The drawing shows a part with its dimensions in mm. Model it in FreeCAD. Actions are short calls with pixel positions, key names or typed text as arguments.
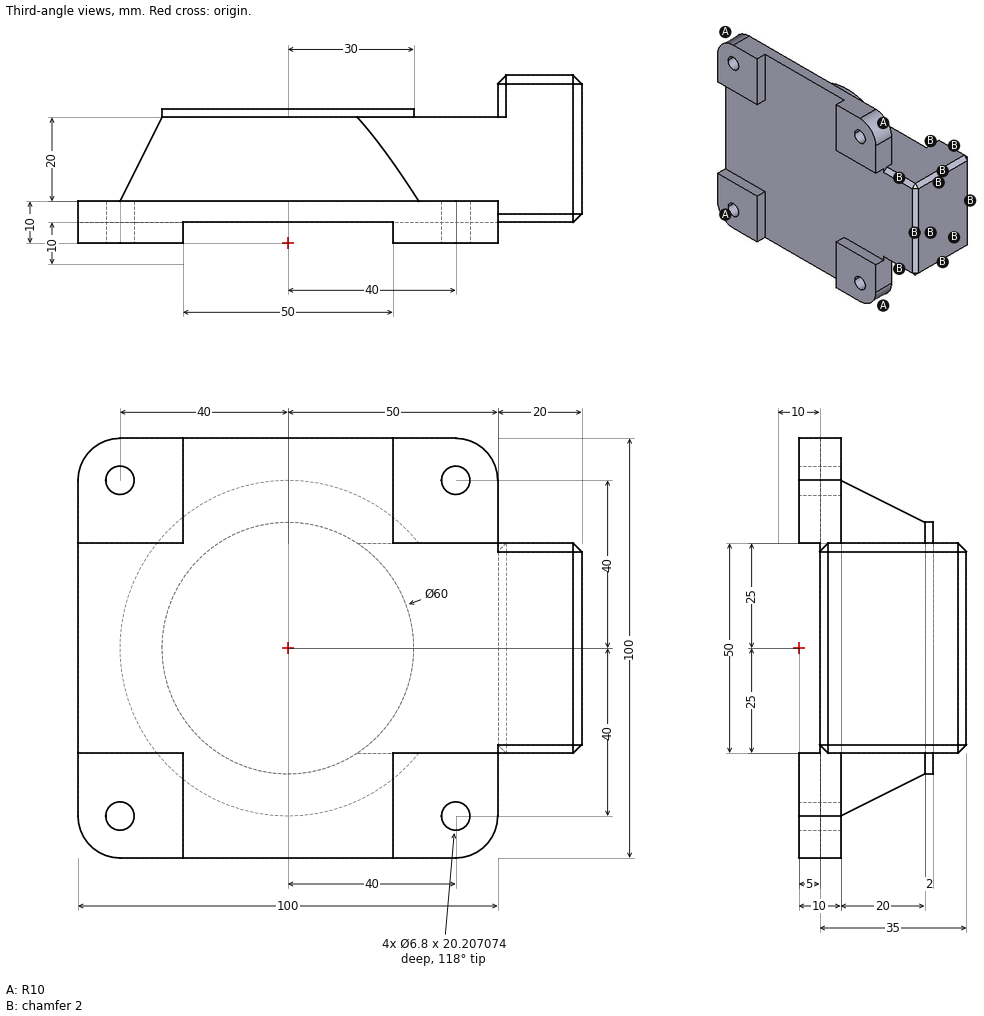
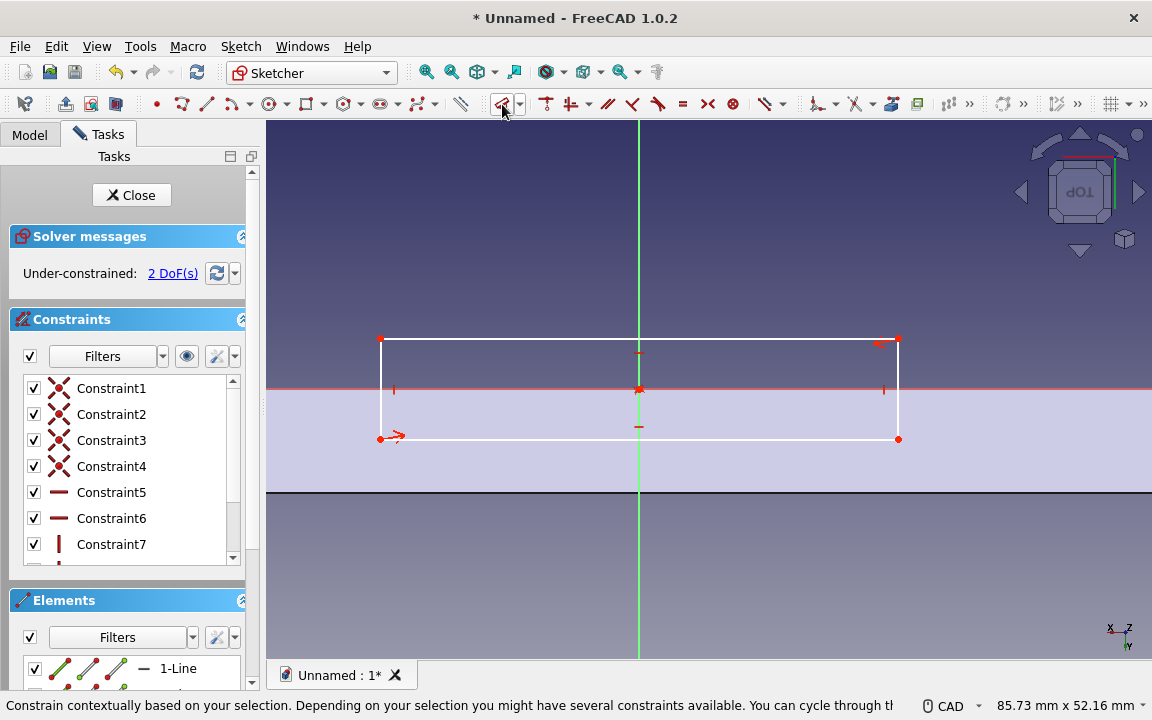
click(536, 440)
click(520, 474)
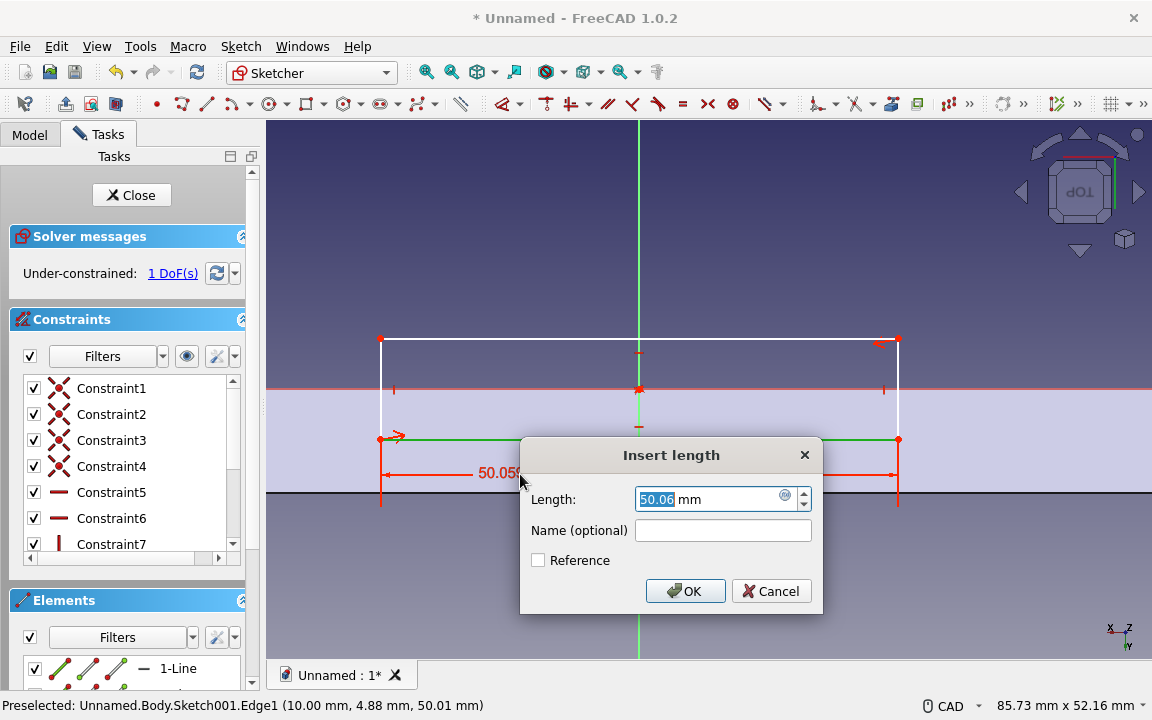
text(50)
key(Return)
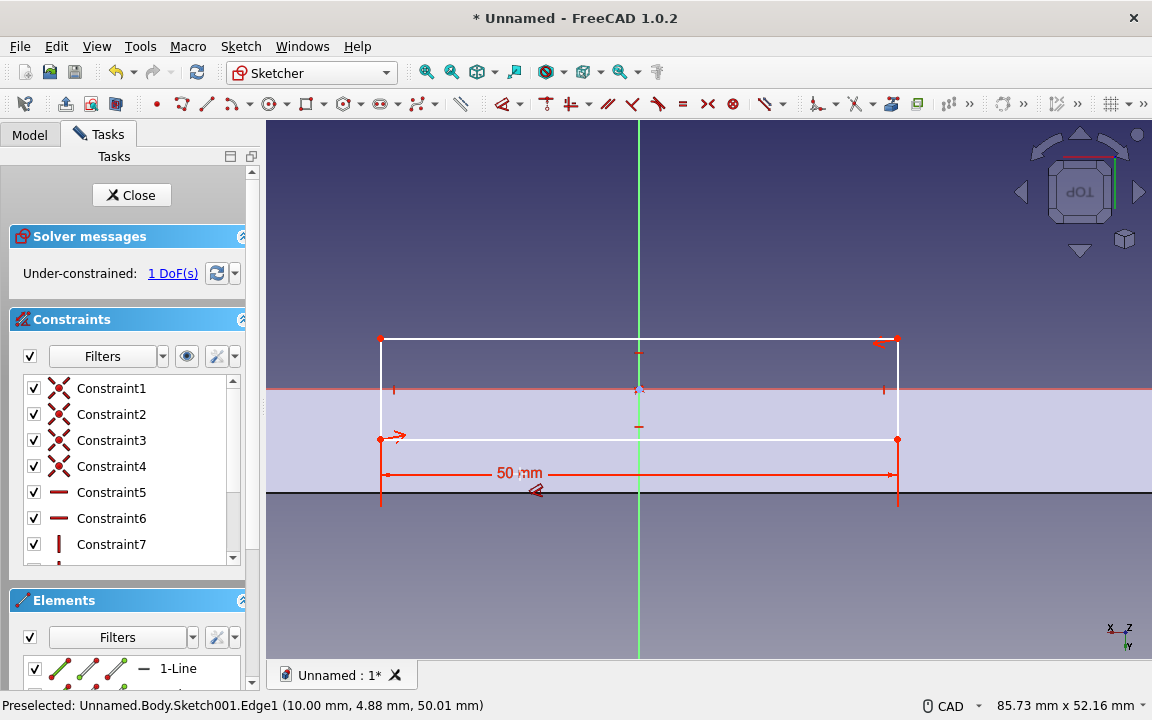
click(898, 410)
click(932, 366)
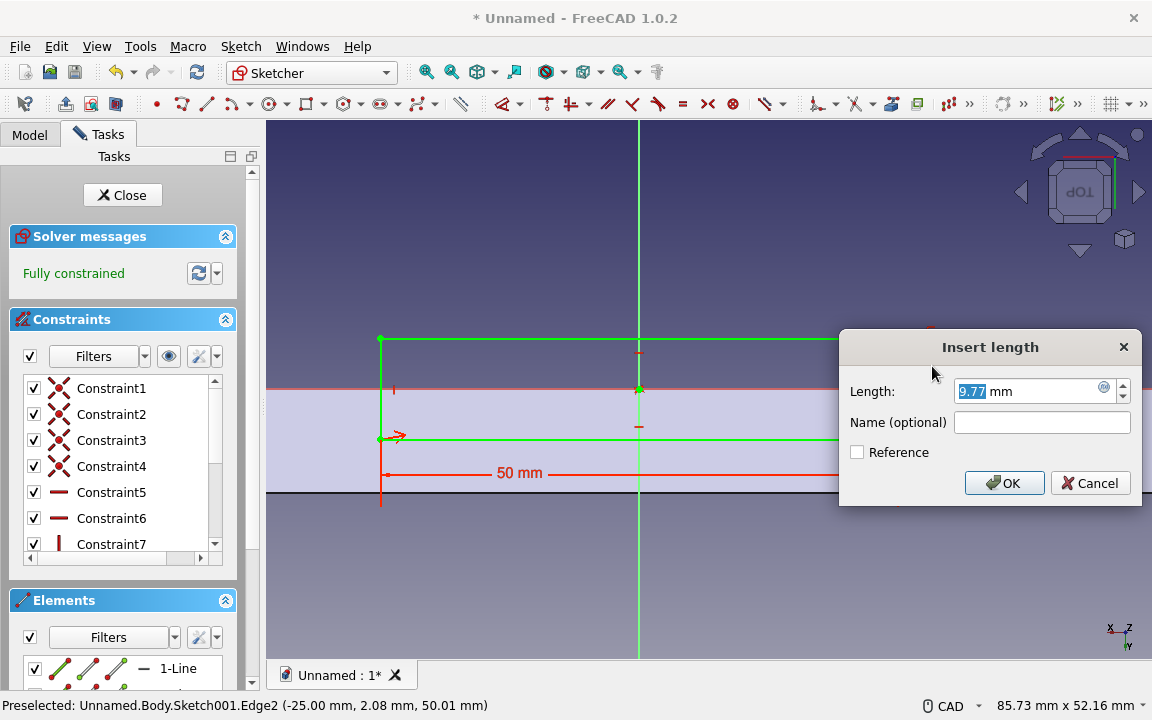
text(10)
key(Return)
key(Escape)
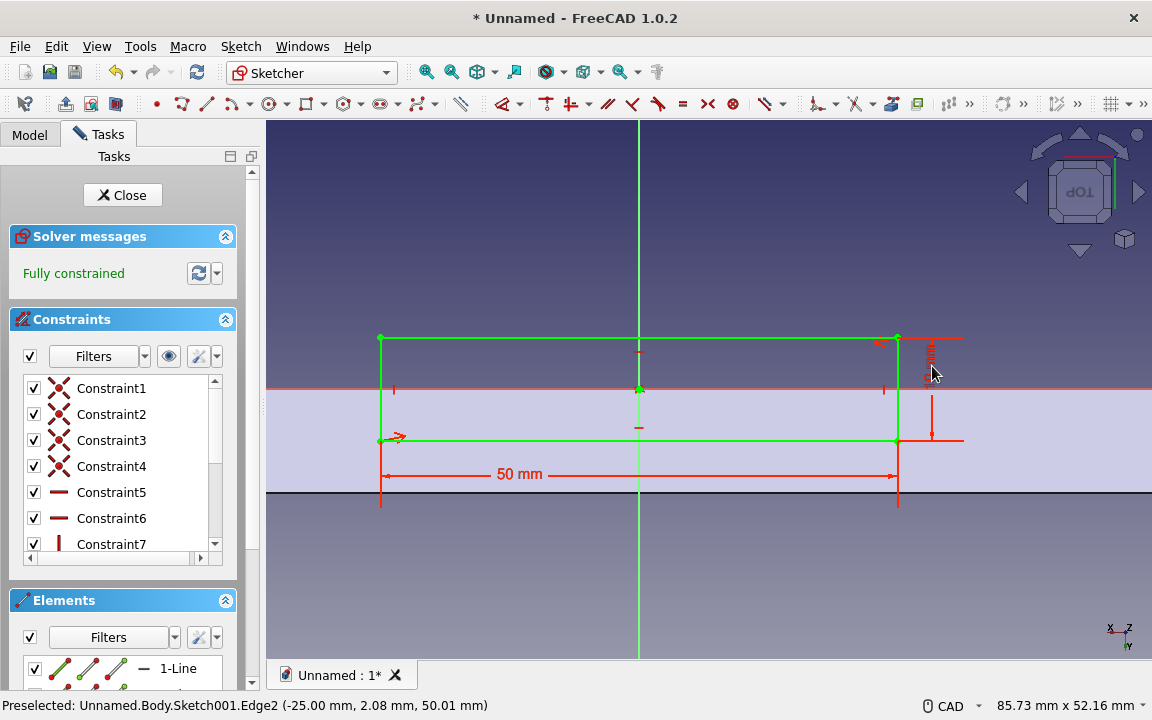
click(123, 195)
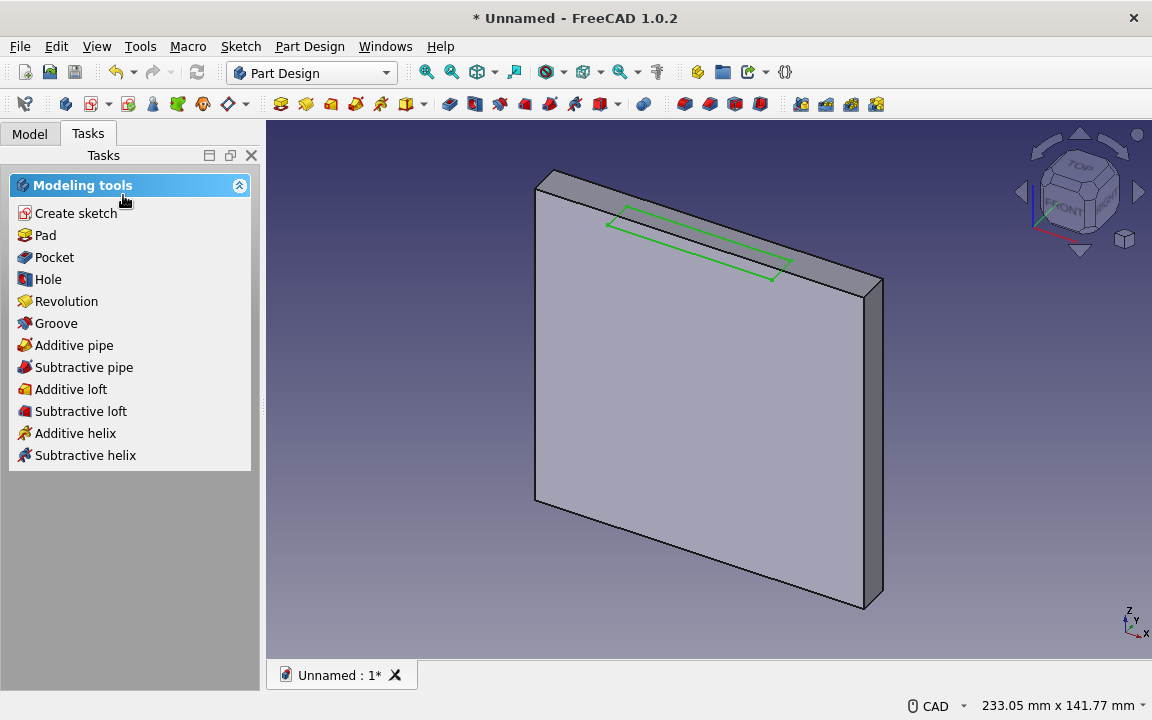
click(450, 104)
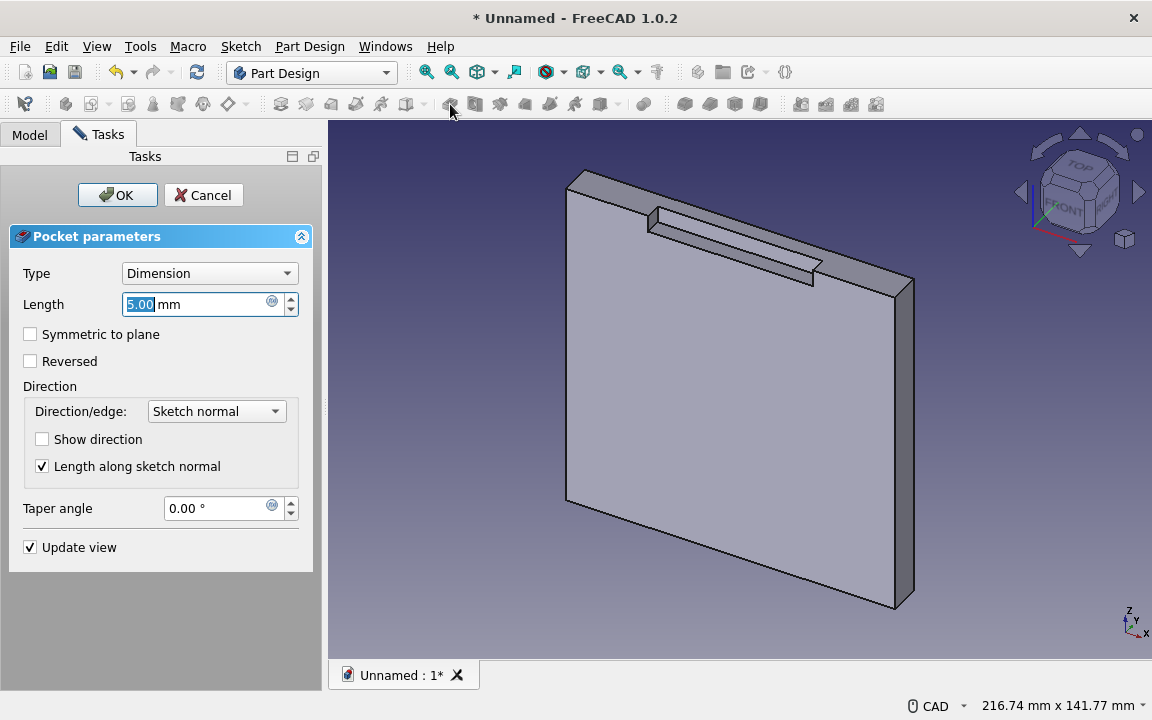
click(210, 274)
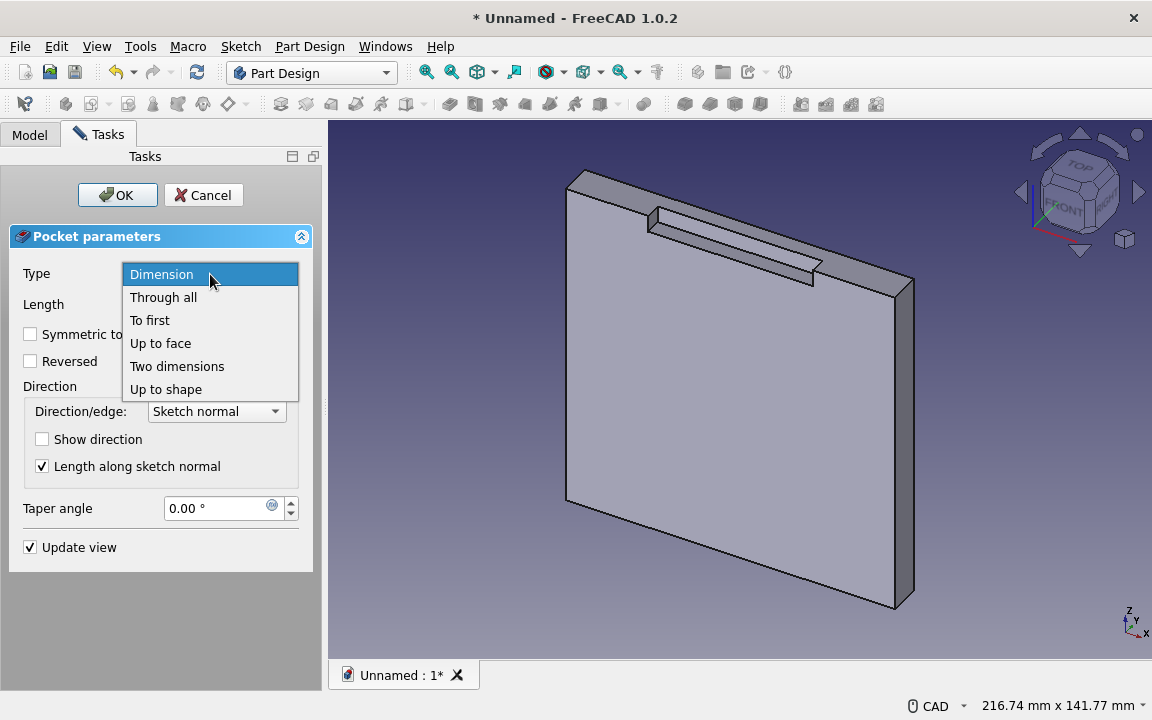
click(208, 298)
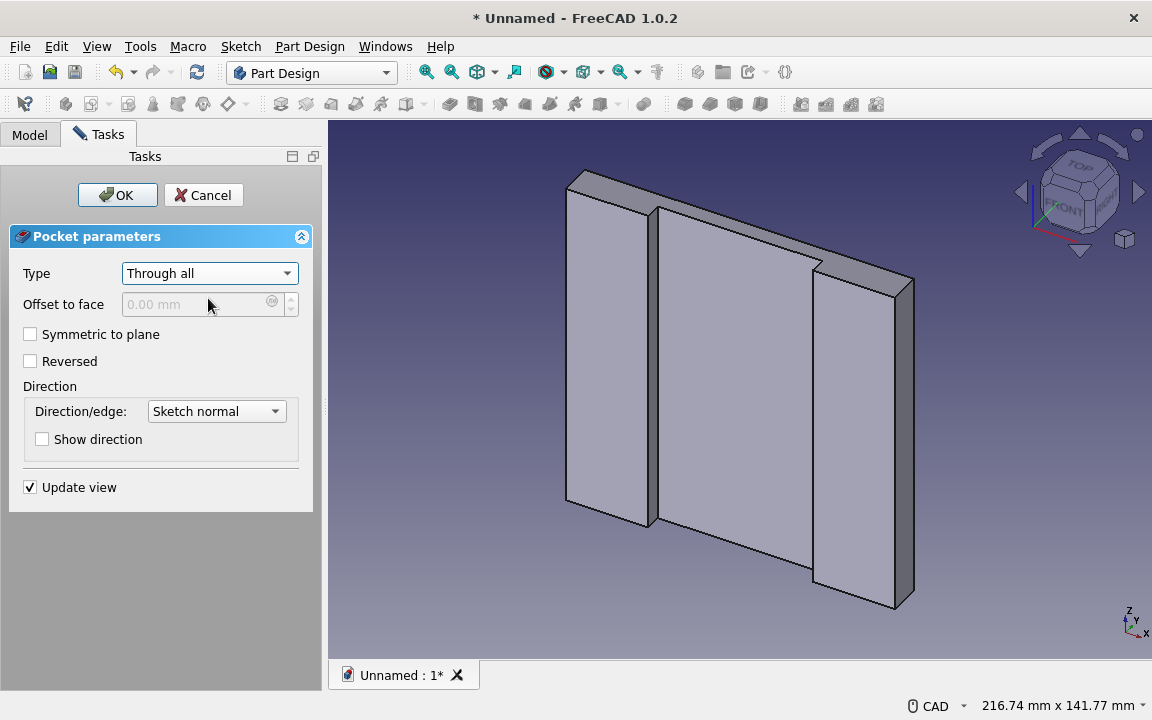
click(118, 195)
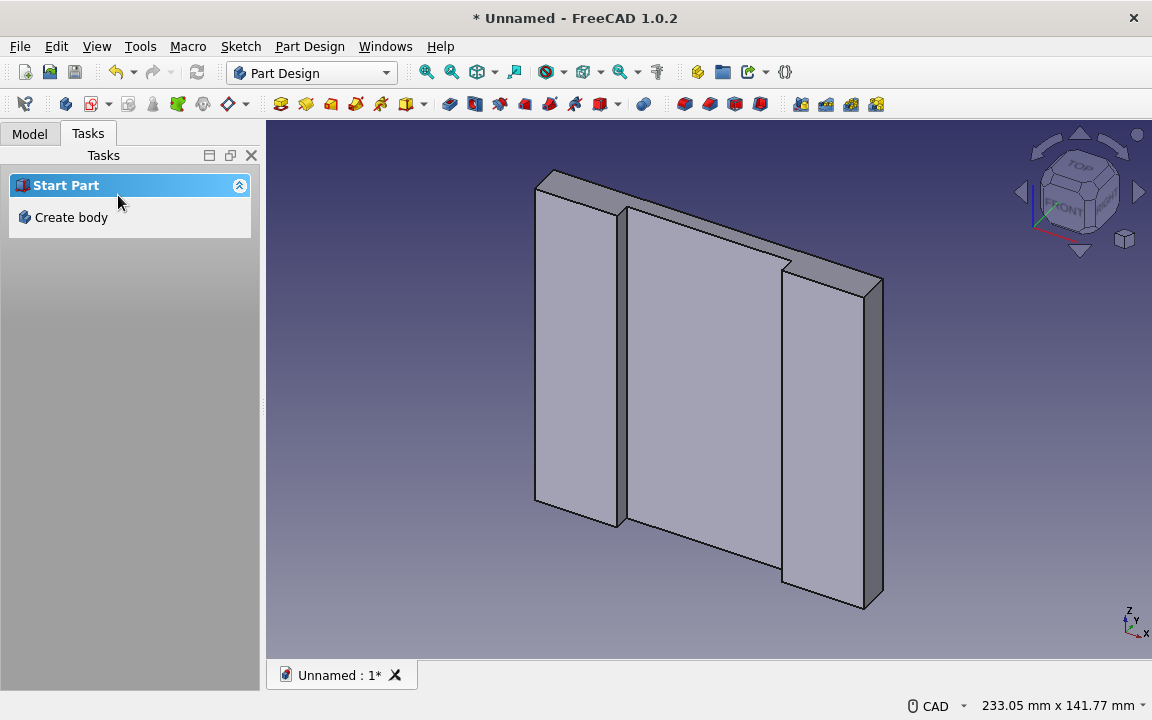
click(874, 310)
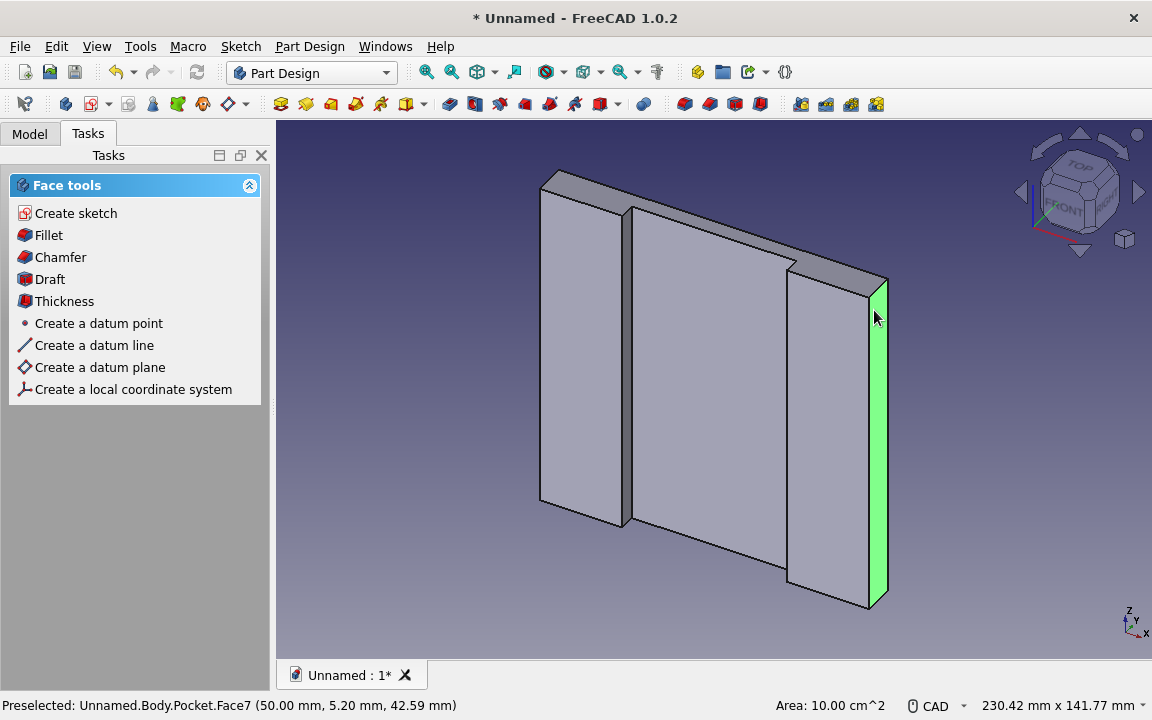
click(90, 104)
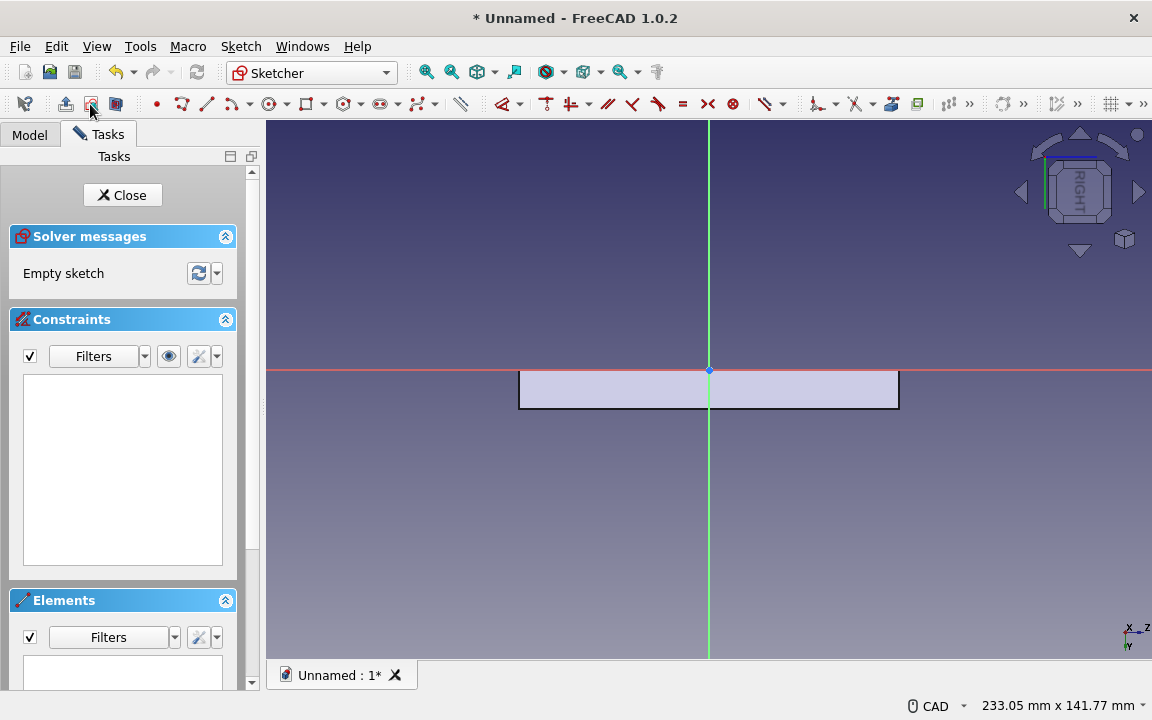
scroll(749, 359, up, 5)